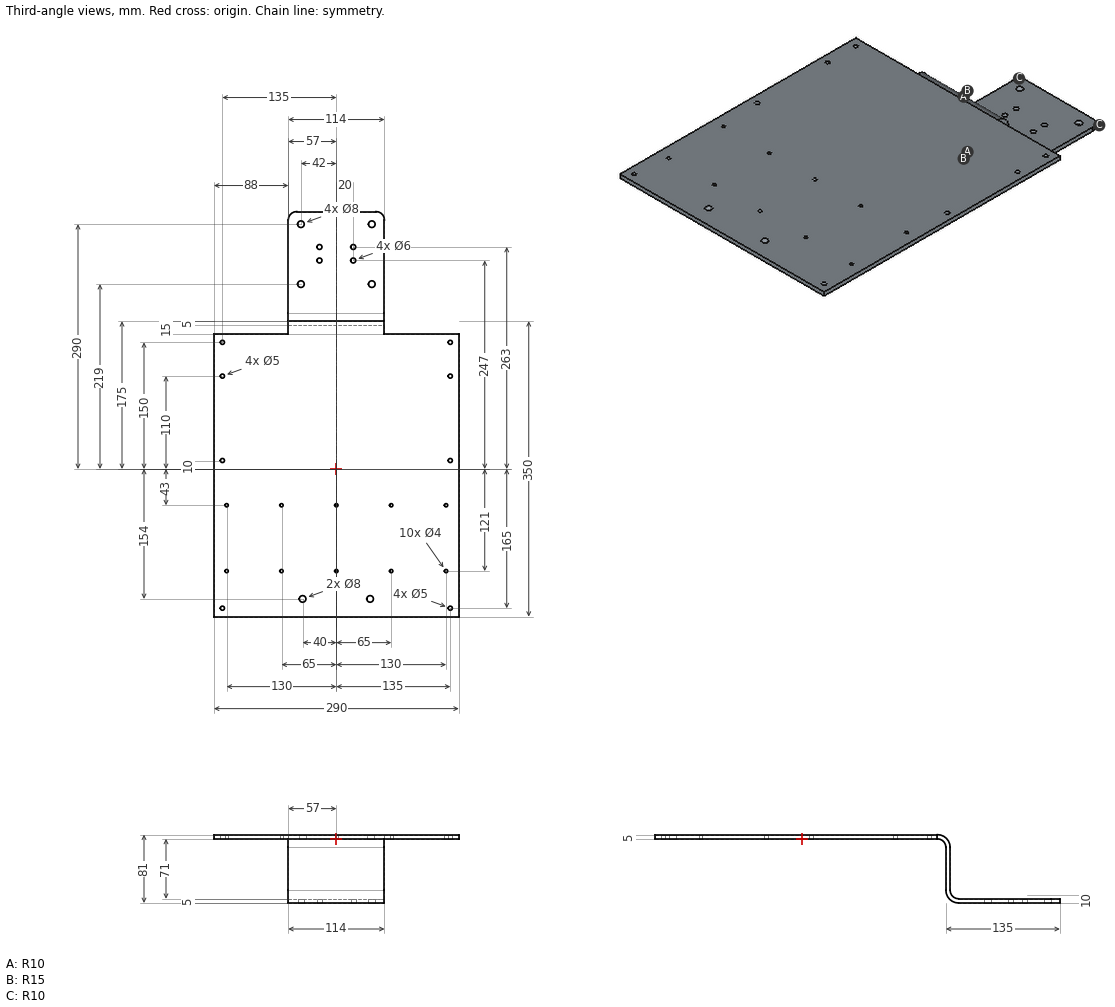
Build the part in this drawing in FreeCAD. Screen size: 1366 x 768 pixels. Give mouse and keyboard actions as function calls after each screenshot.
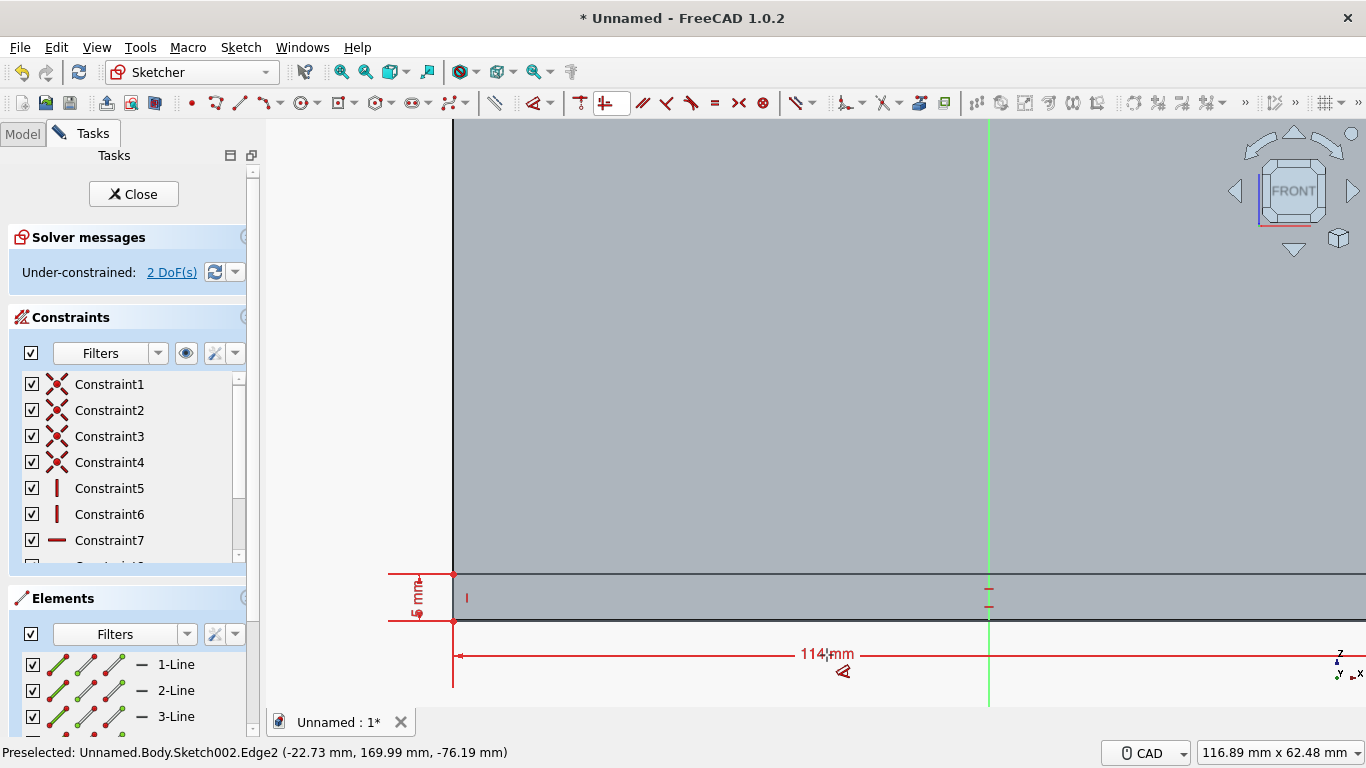
click(453, 574)
click(721, 608)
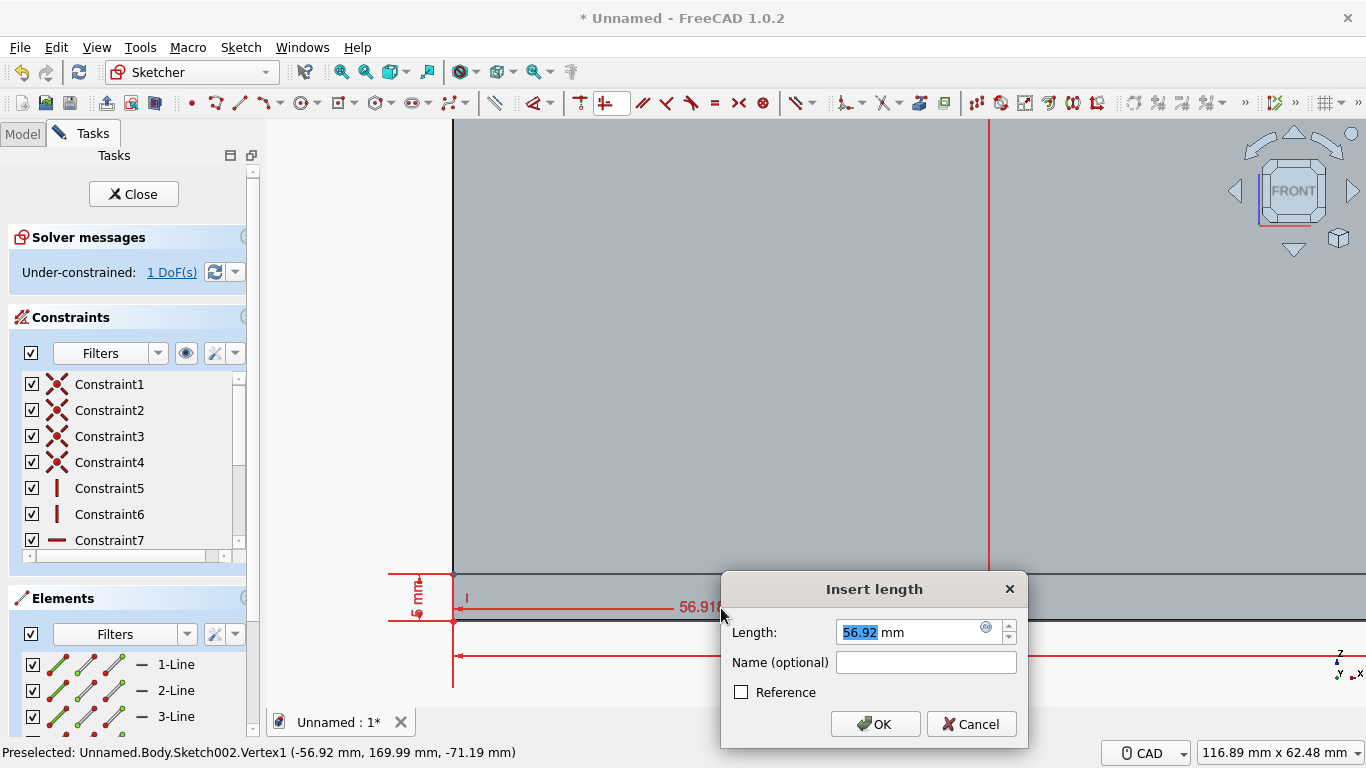
text(57)
key(Return)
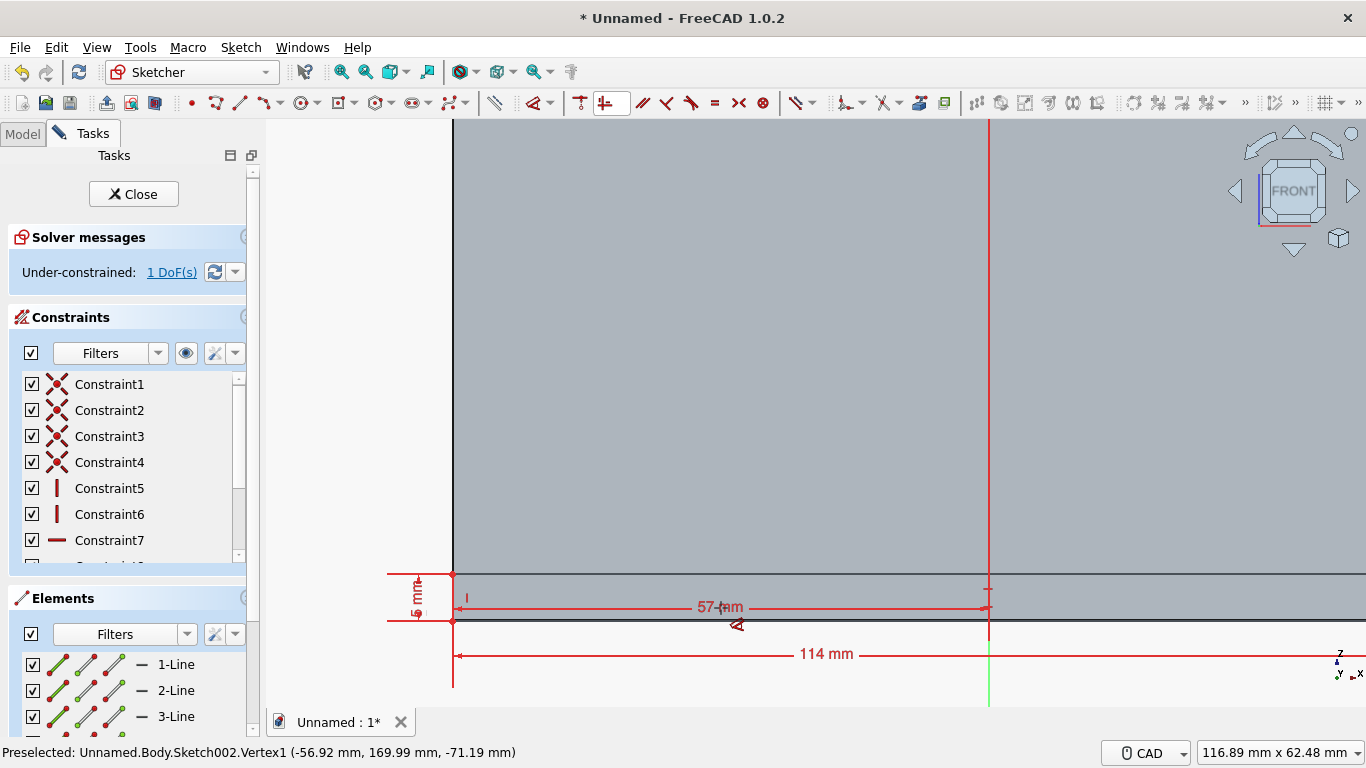
click(453, 574)
click(419, 361)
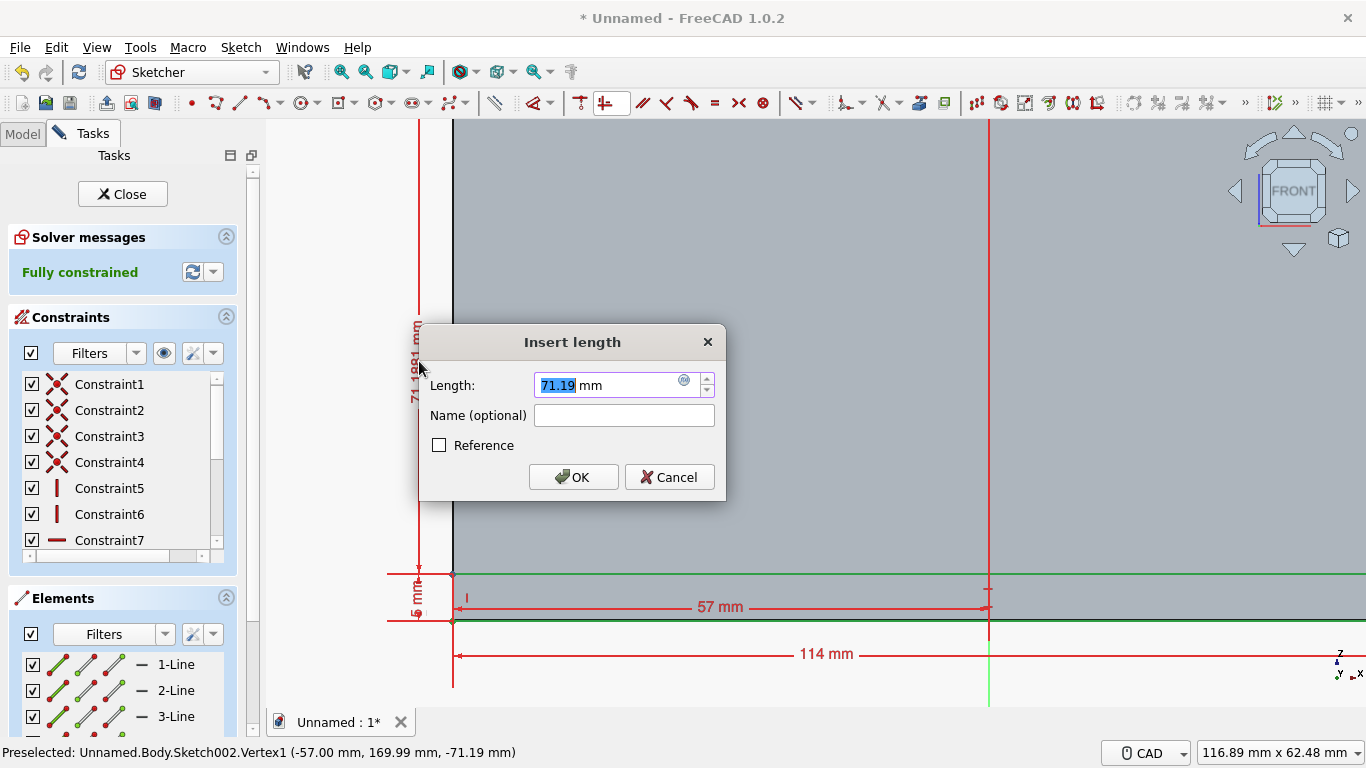
text(71)
key(Return)
key(Escape)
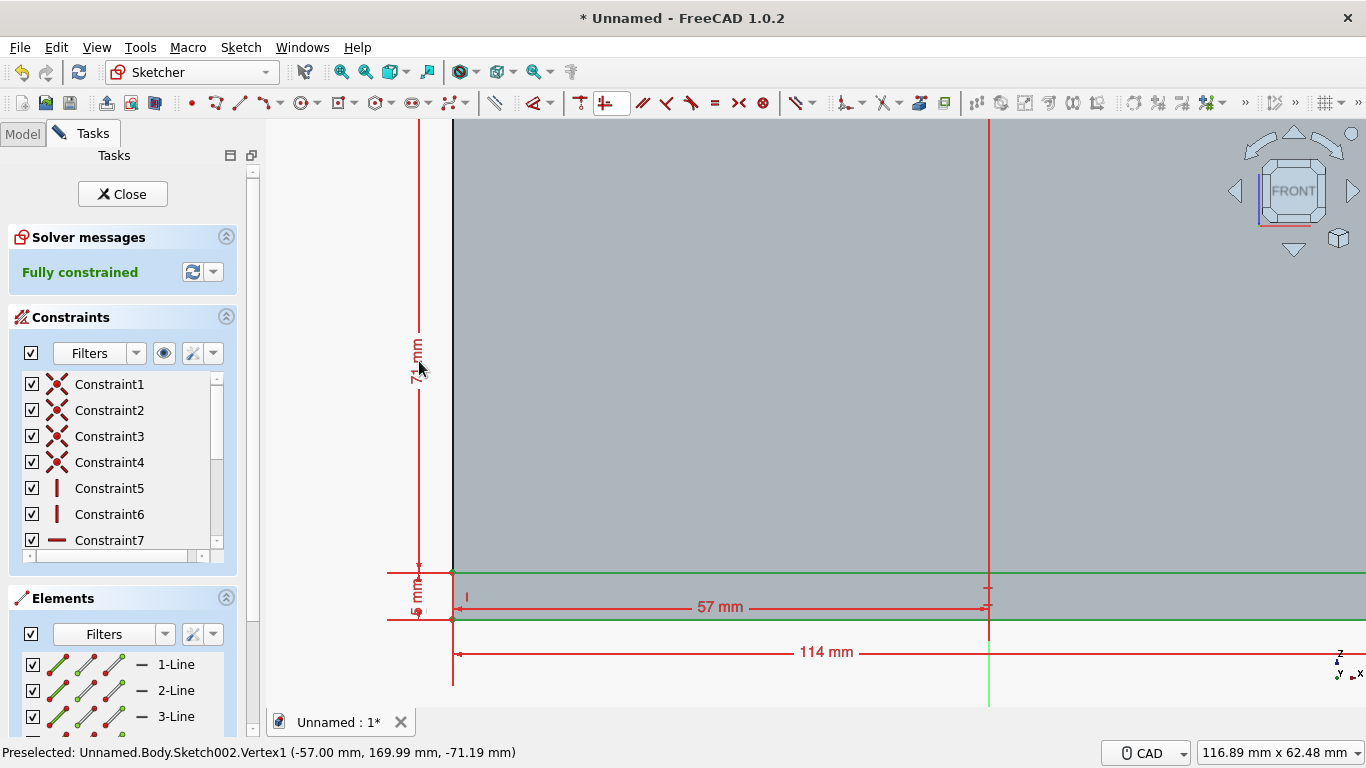
click(123, 194)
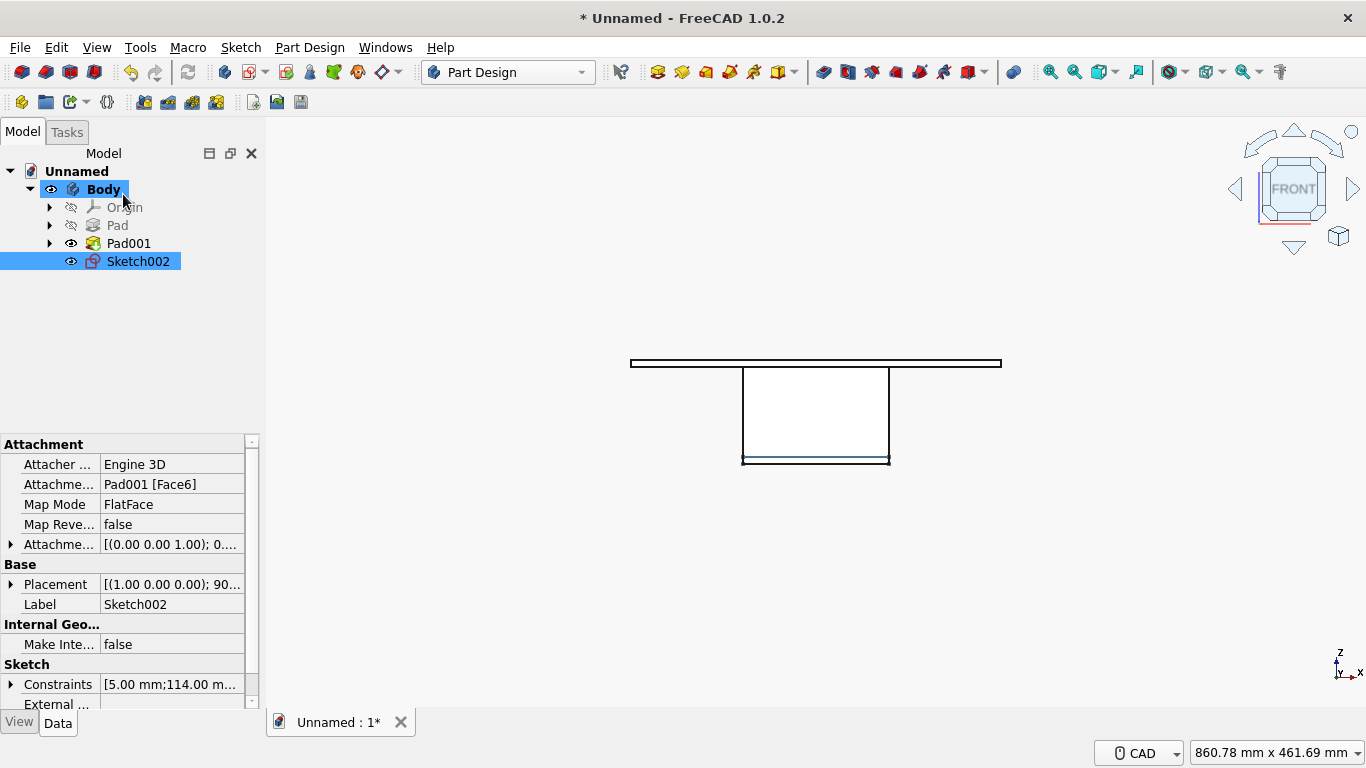
click(658, 72)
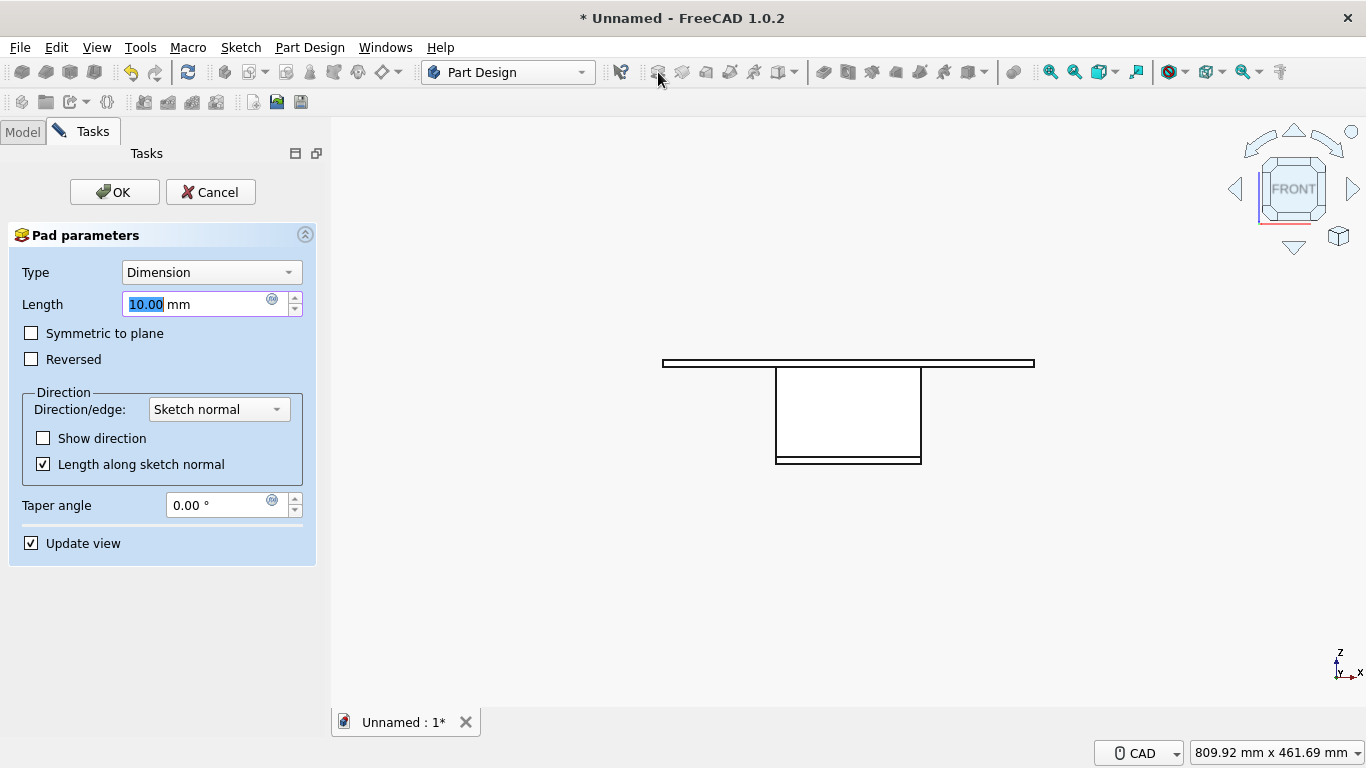
text(135)
key(Tab)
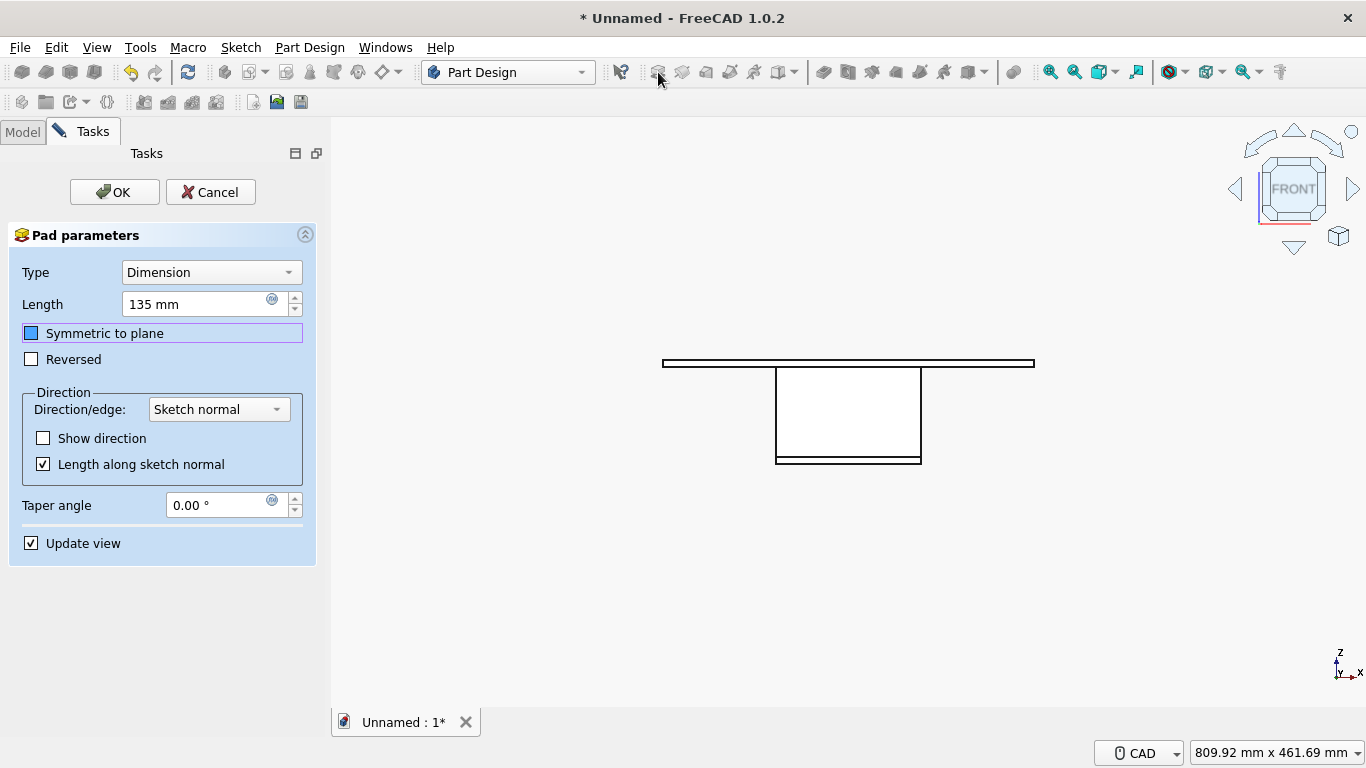
click(30, 359)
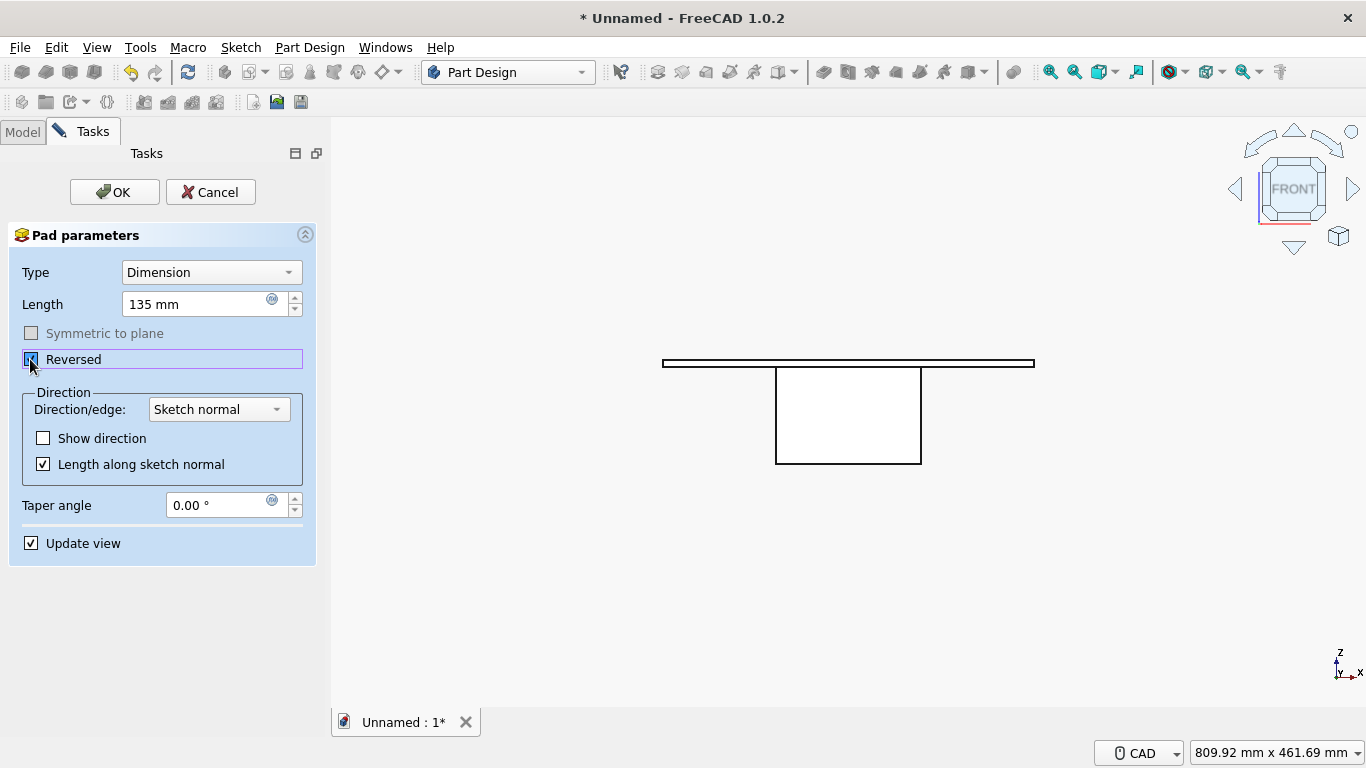
click(115, 192)